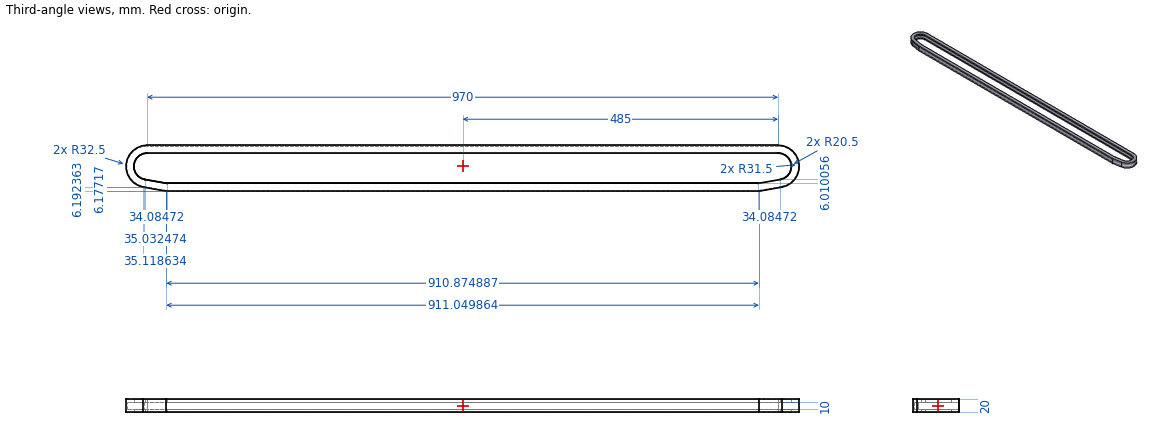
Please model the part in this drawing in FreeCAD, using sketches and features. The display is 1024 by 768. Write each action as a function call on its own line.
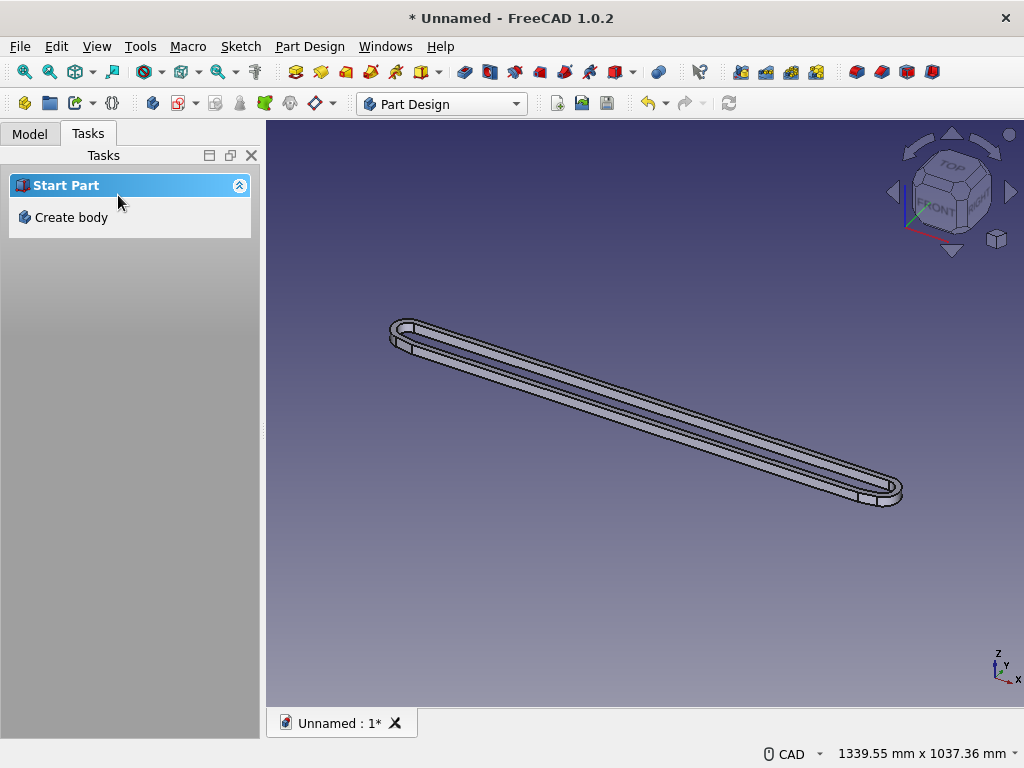
click(178, 104)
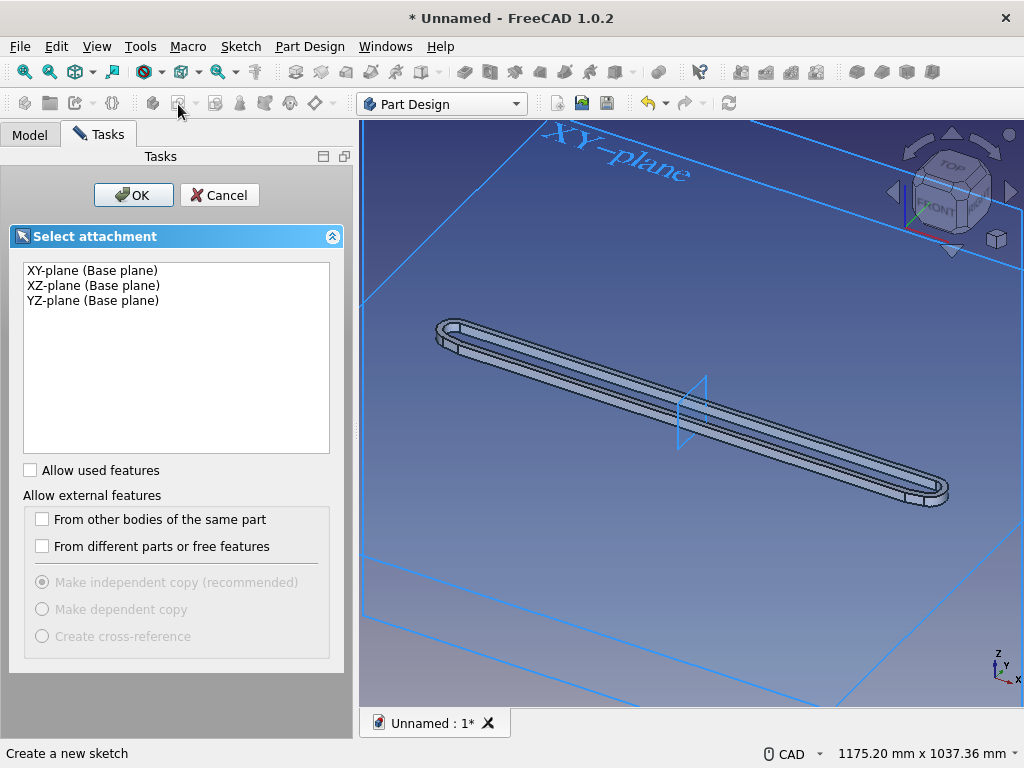
click(84, 270)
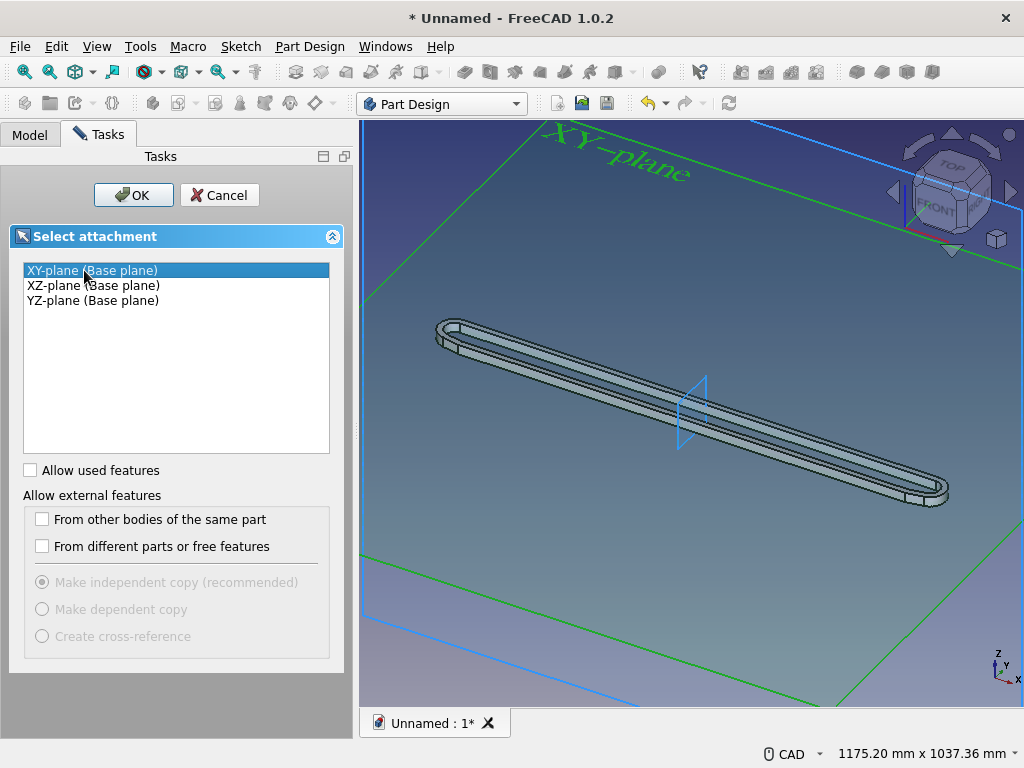
click(134, 195)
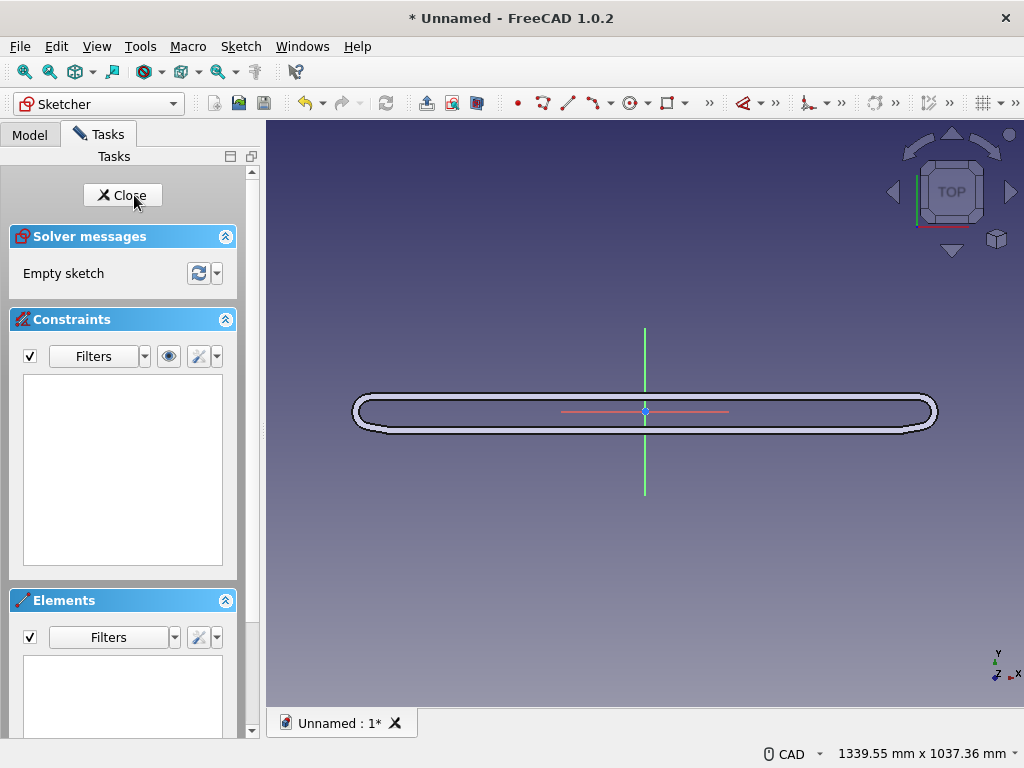
key(q)
key(s)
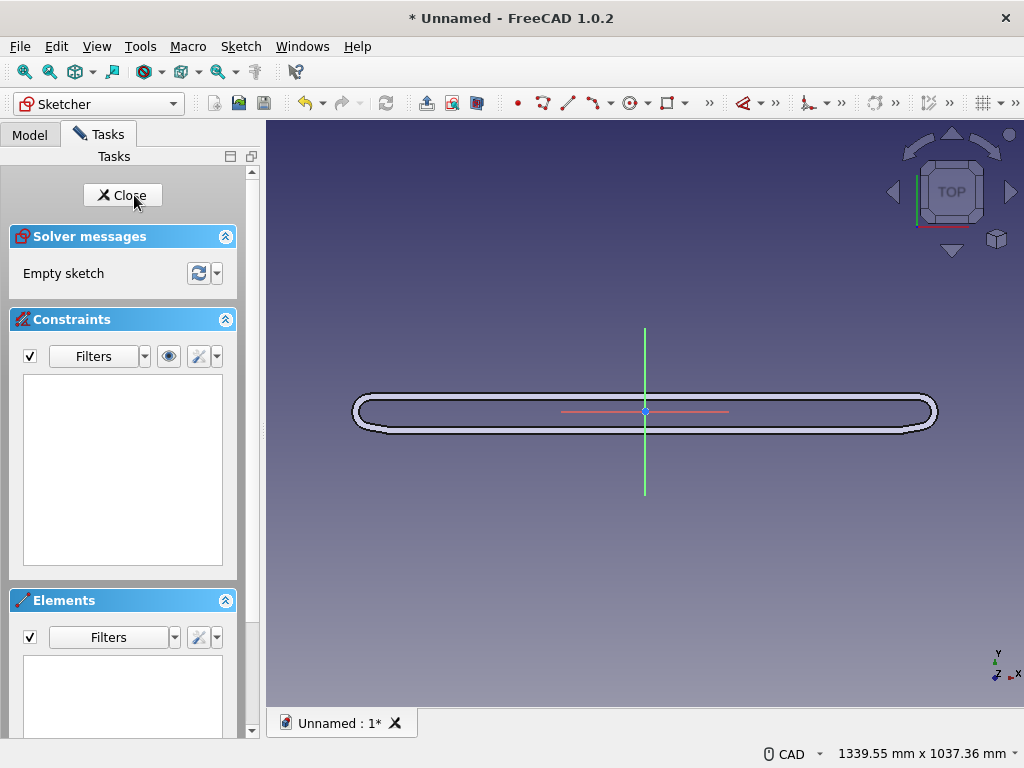
scroll(437, 413, down, 2)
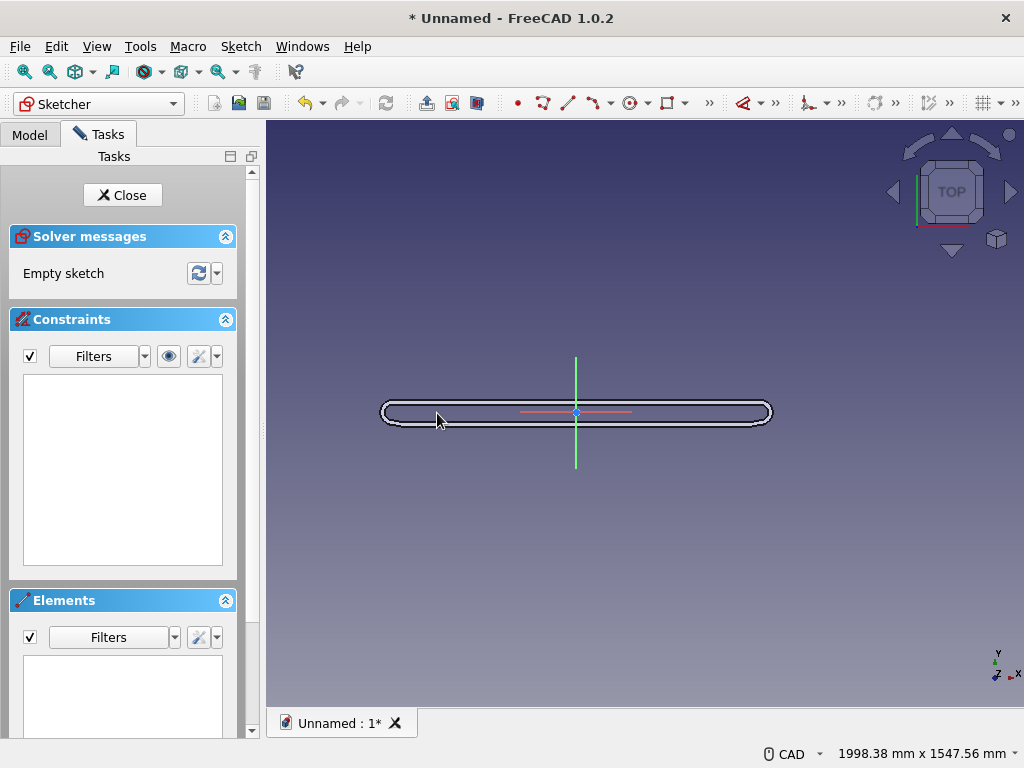
key(g)
key(l)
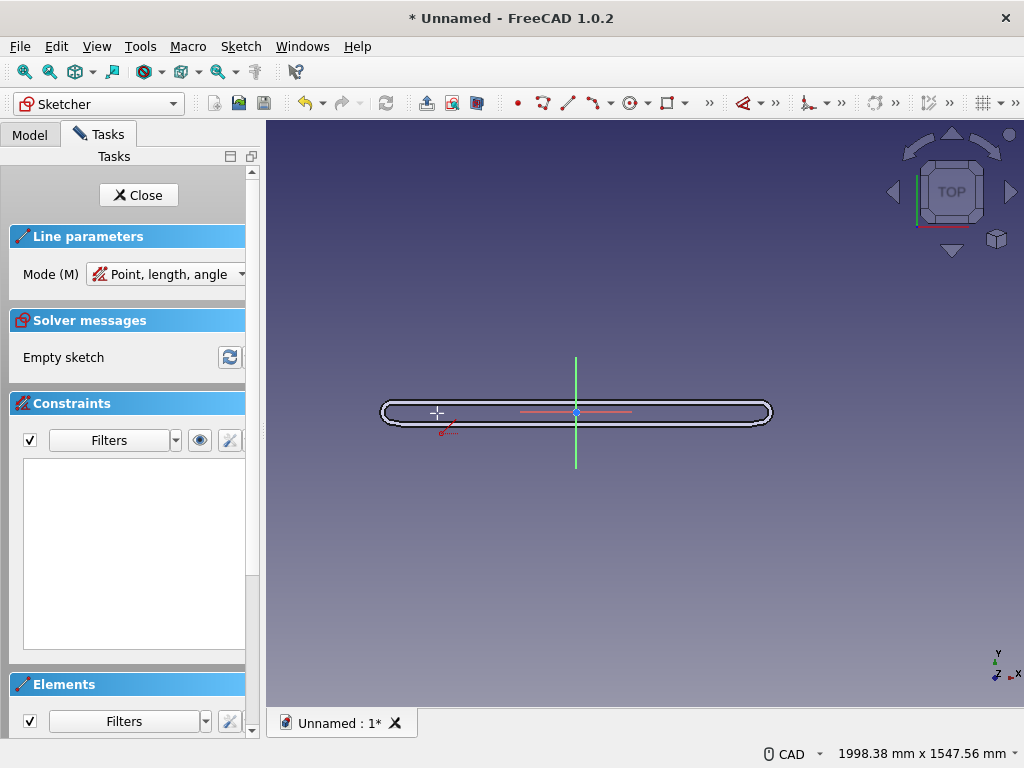
scroll(760, 400, up, 2)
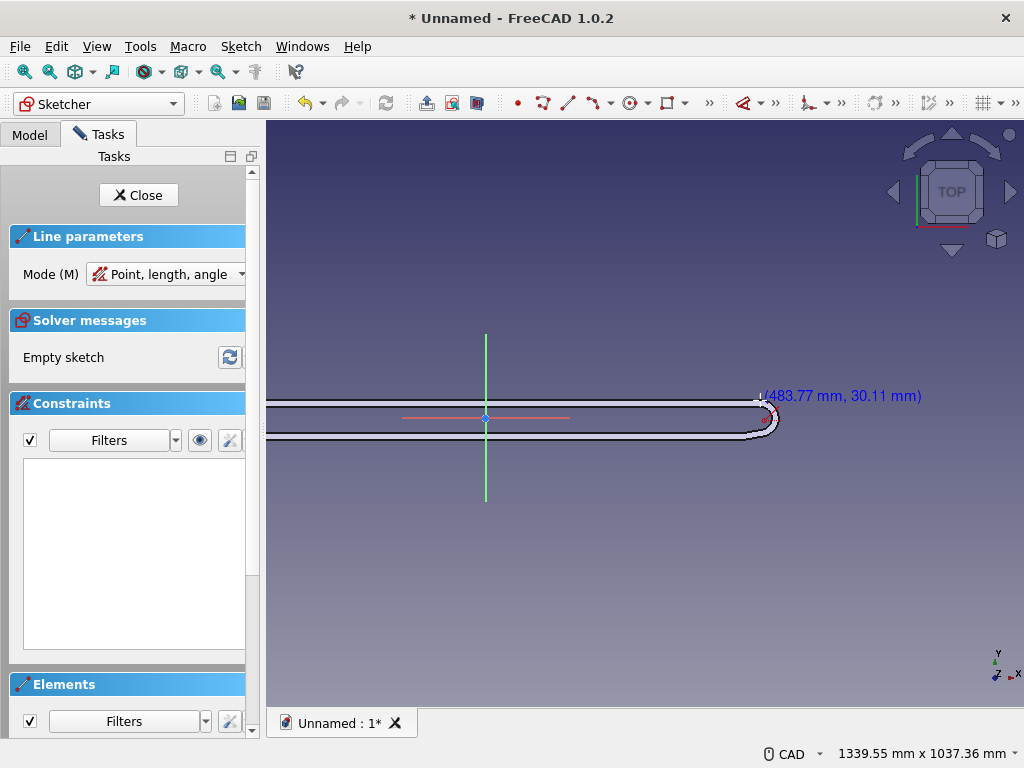
click(760, 400)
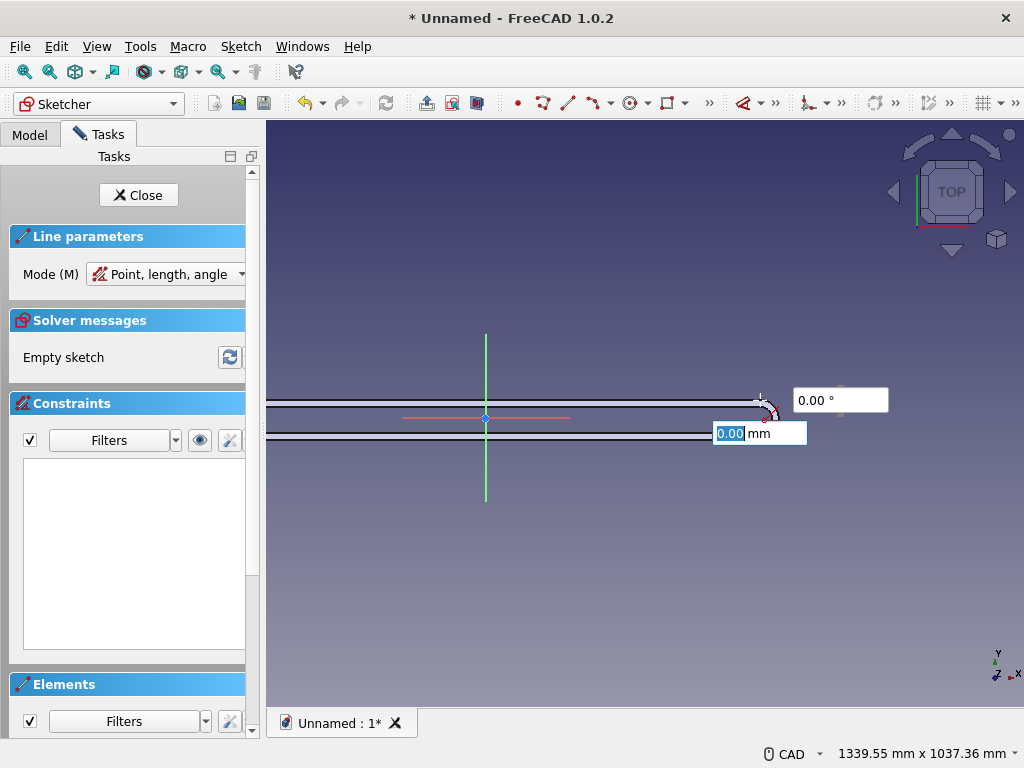
scroll(761, 400, down, 2)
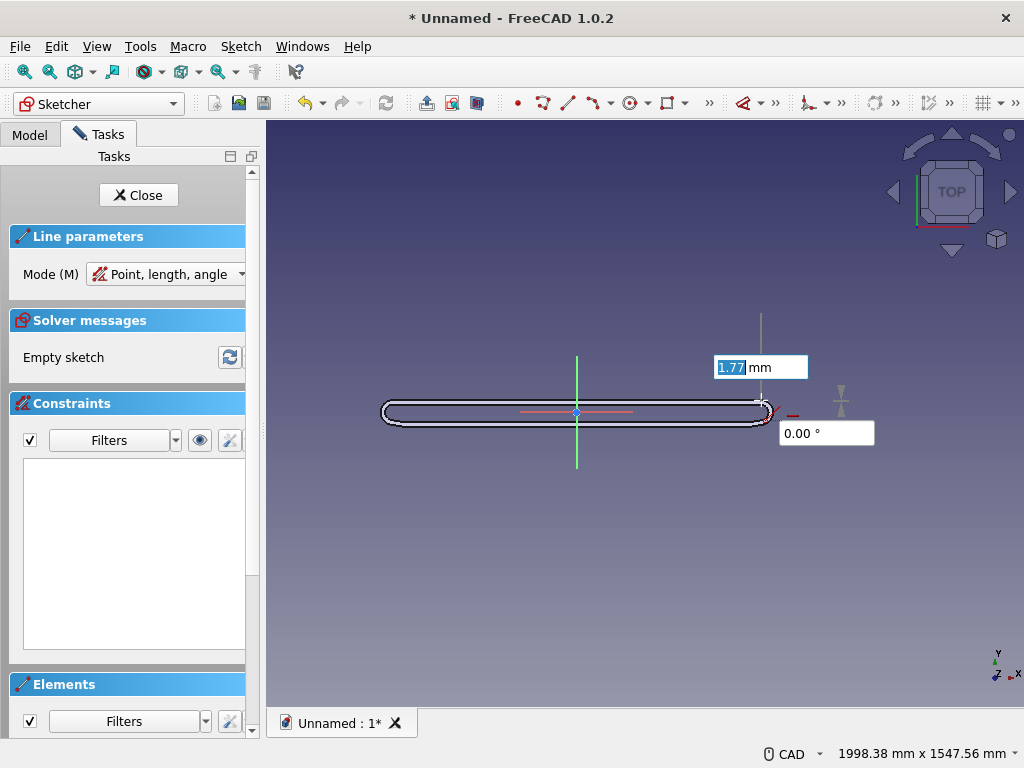
scroll(393, 400, up, 2)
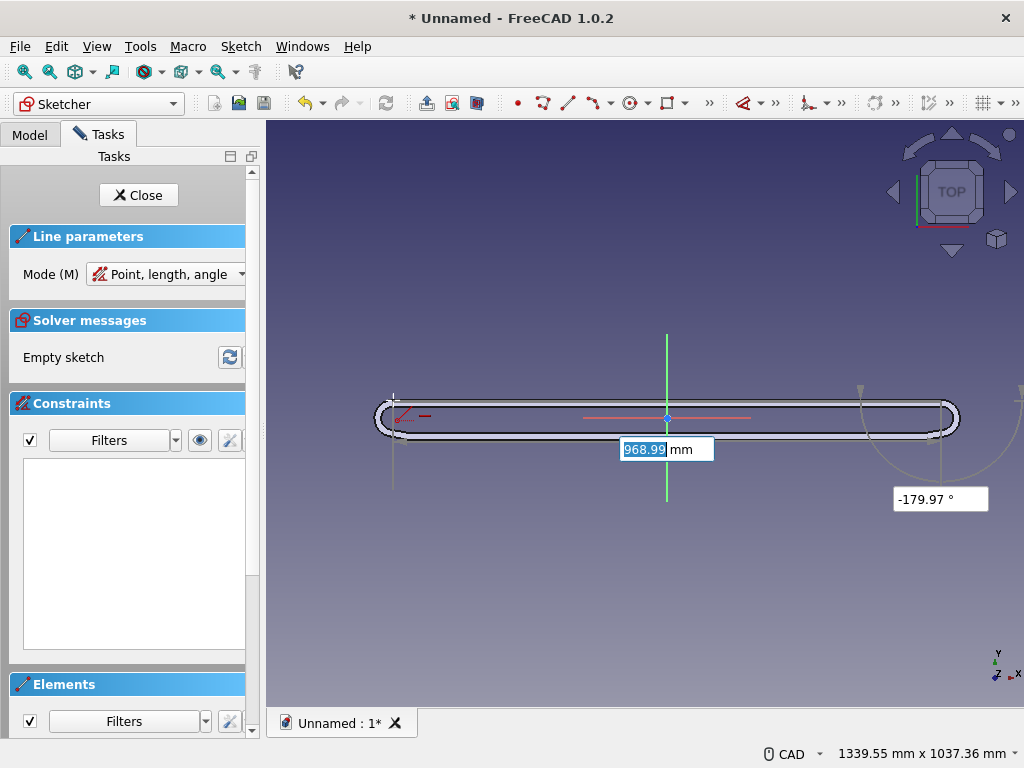
click(393, 400)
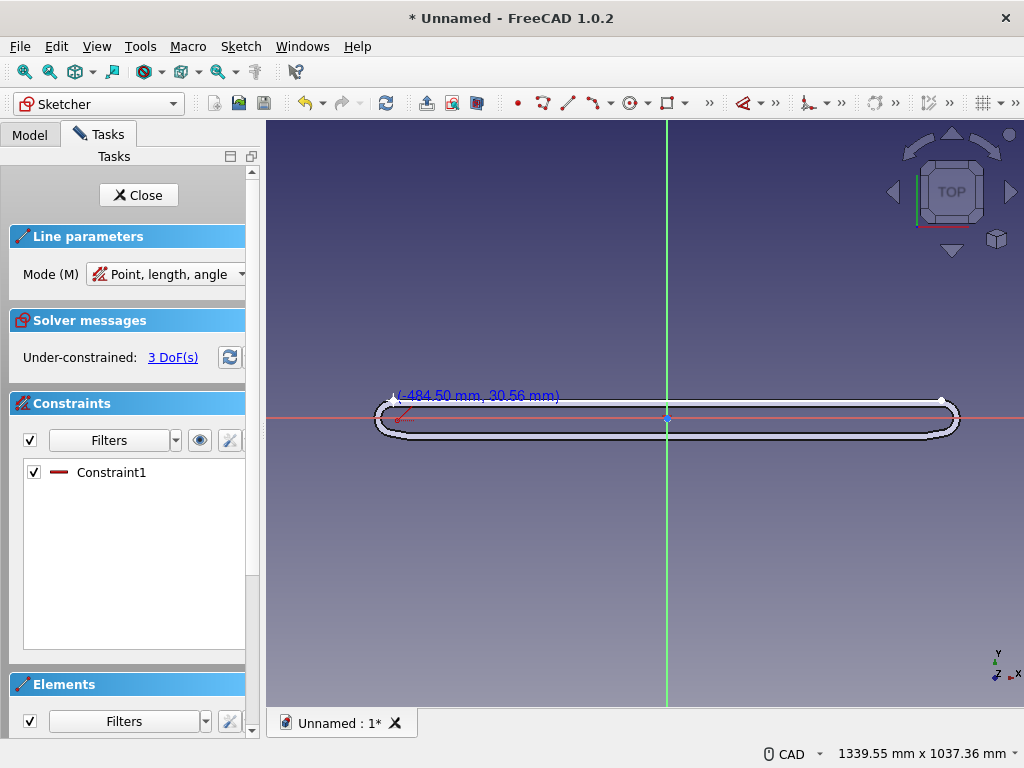
key(g)
key(m)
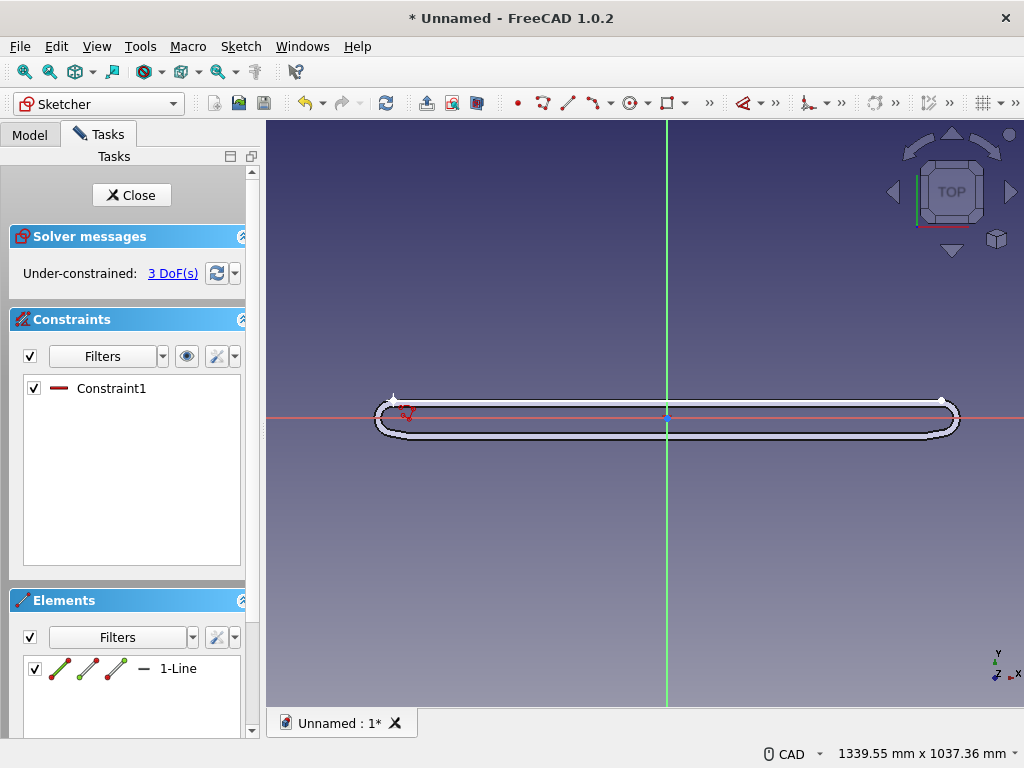
click(390, 436)
click(409, 439)